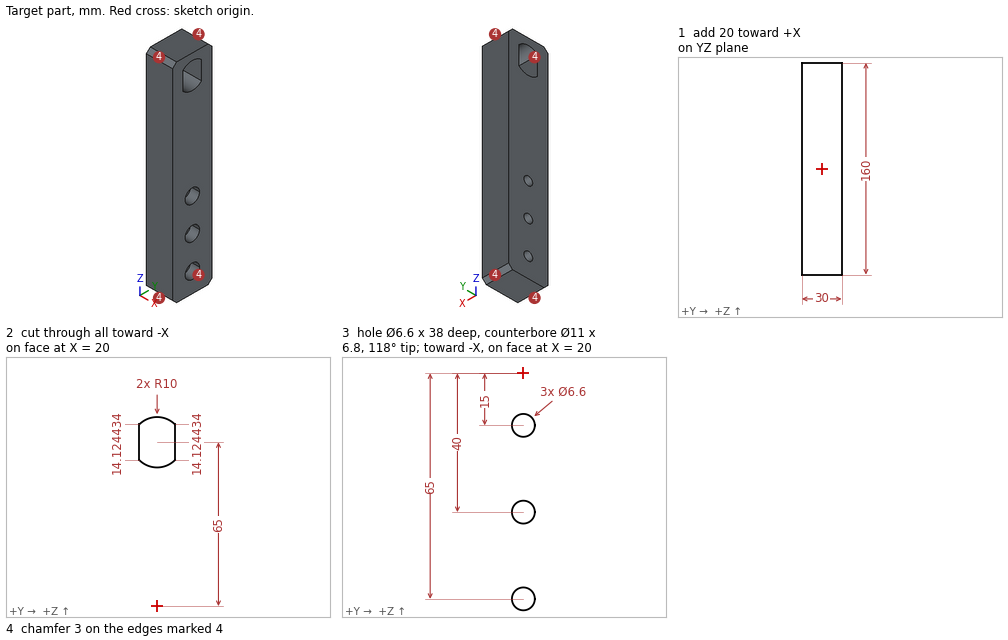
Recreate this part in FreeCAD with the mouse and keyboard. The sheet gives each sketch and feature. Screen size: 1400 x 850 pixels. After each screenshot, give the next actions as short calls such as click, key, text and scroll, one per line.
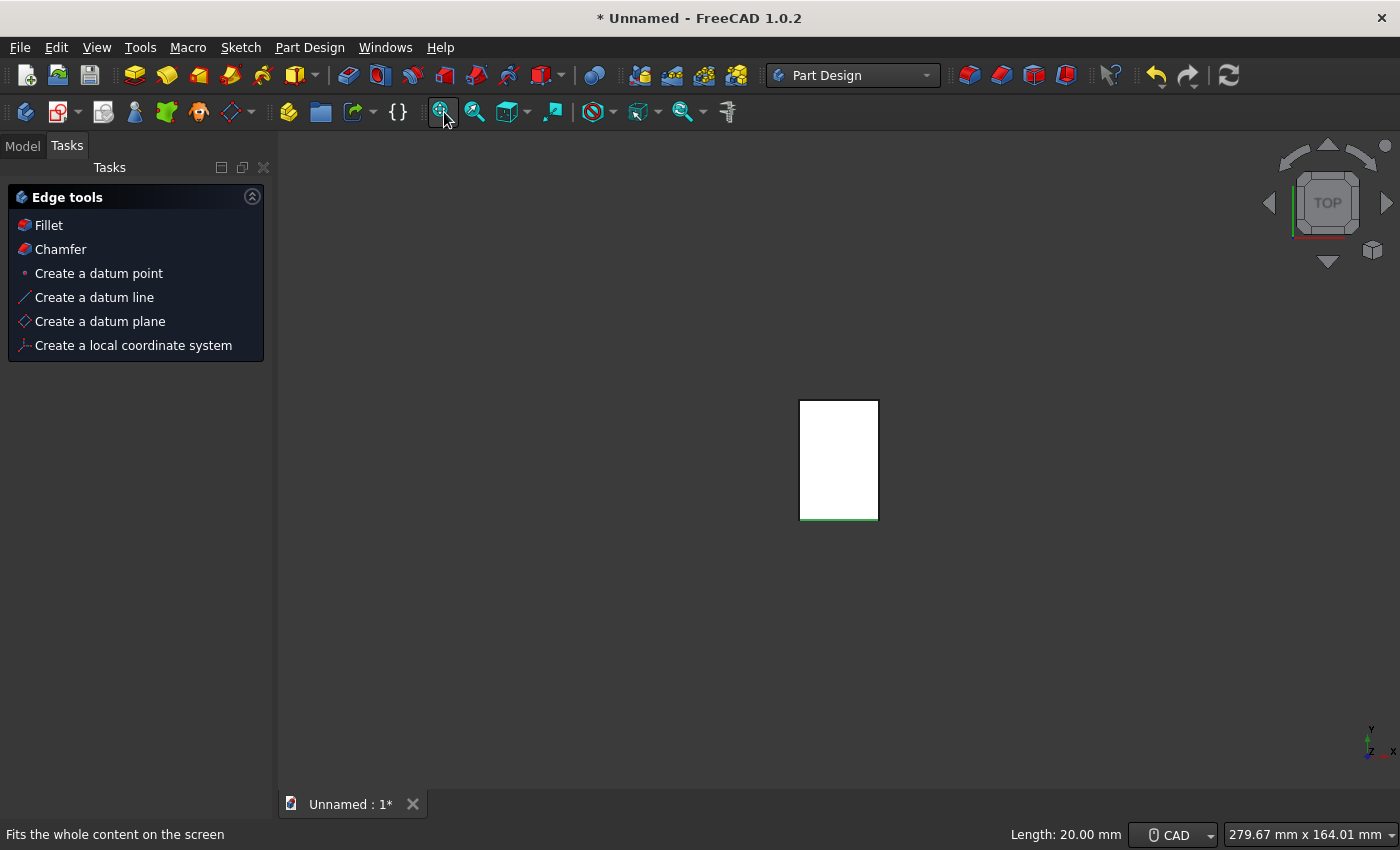
click(839, 399, ctrl)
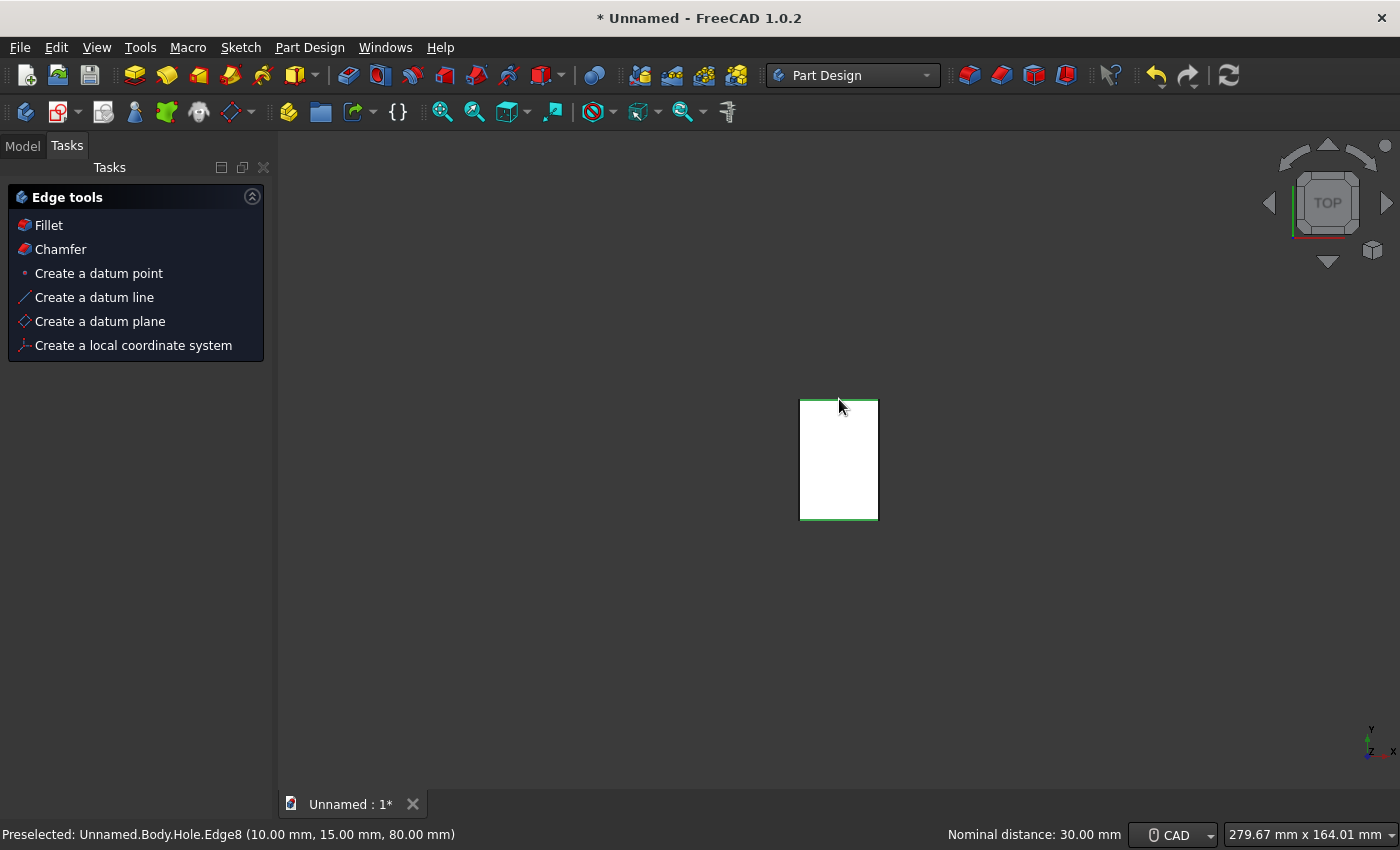
key(1)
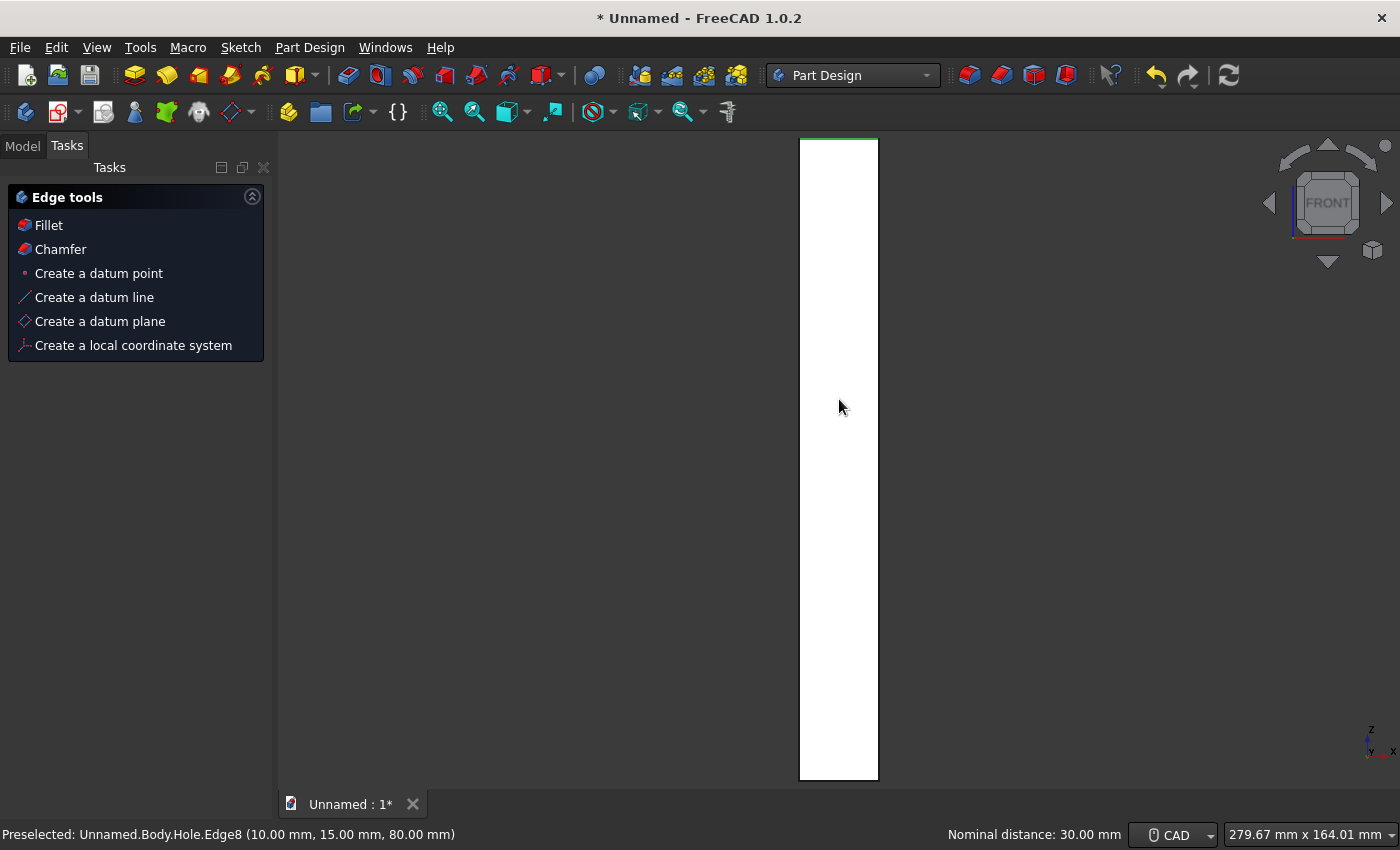
key(3)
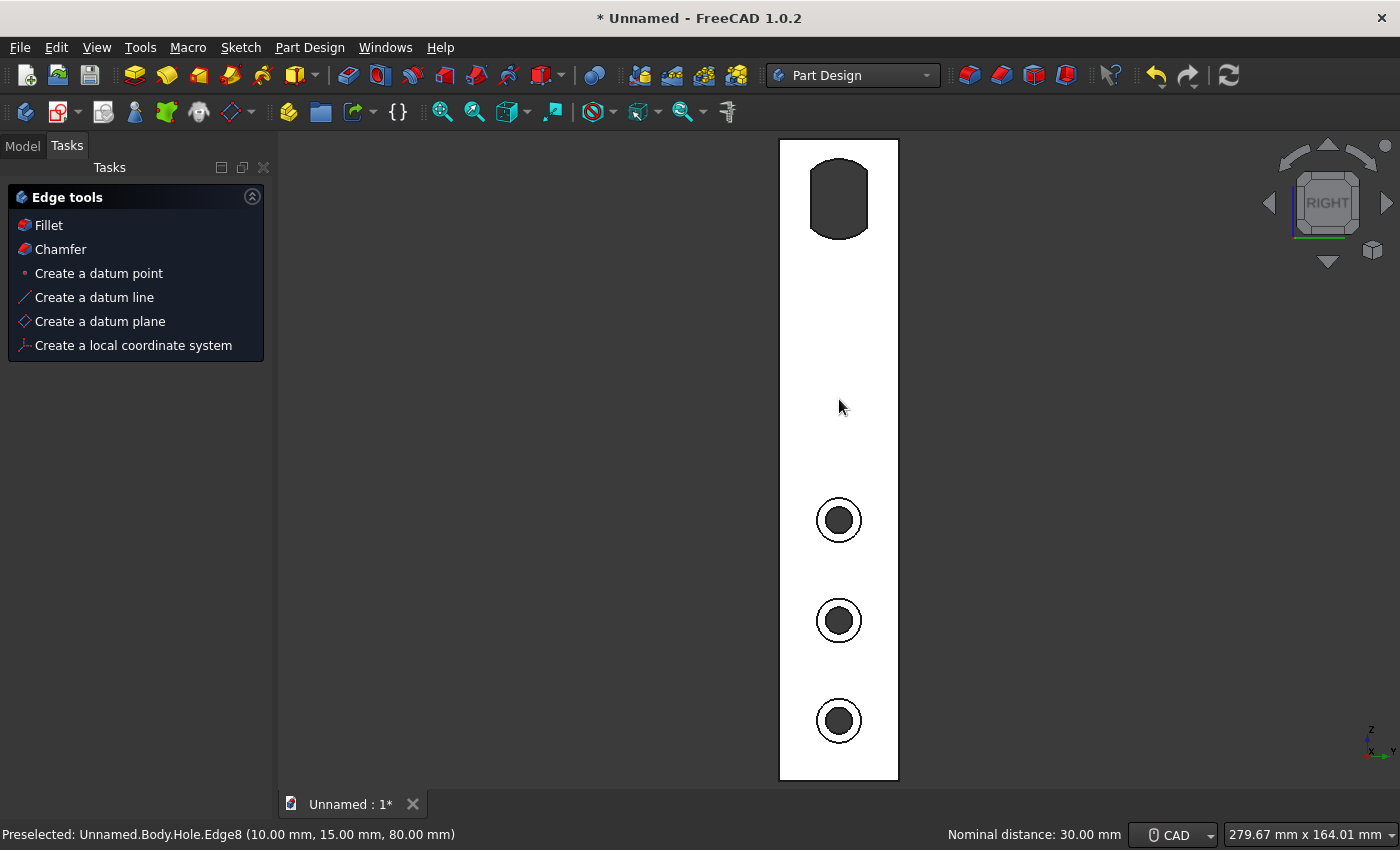
key(5)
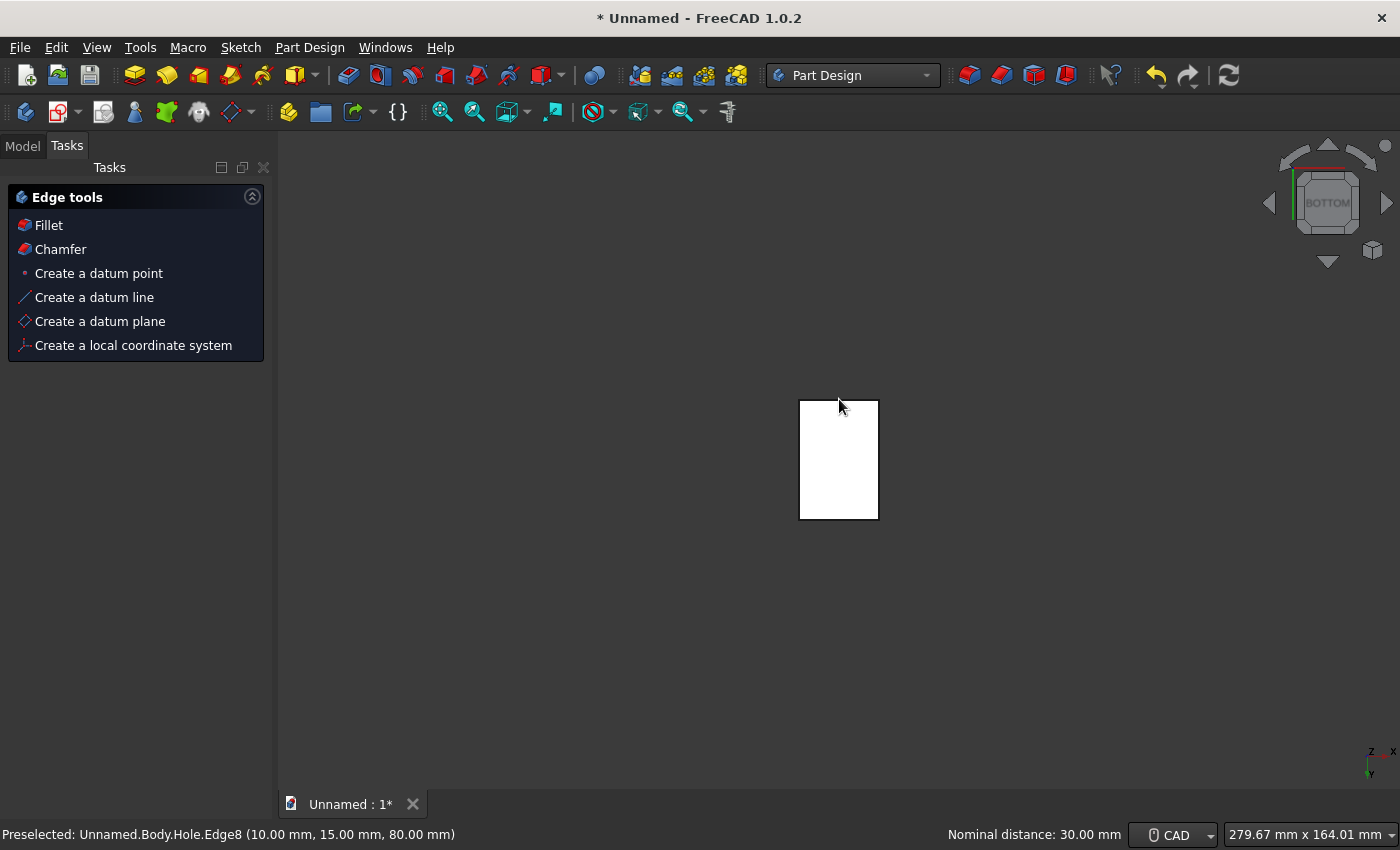
key(v)
key(f)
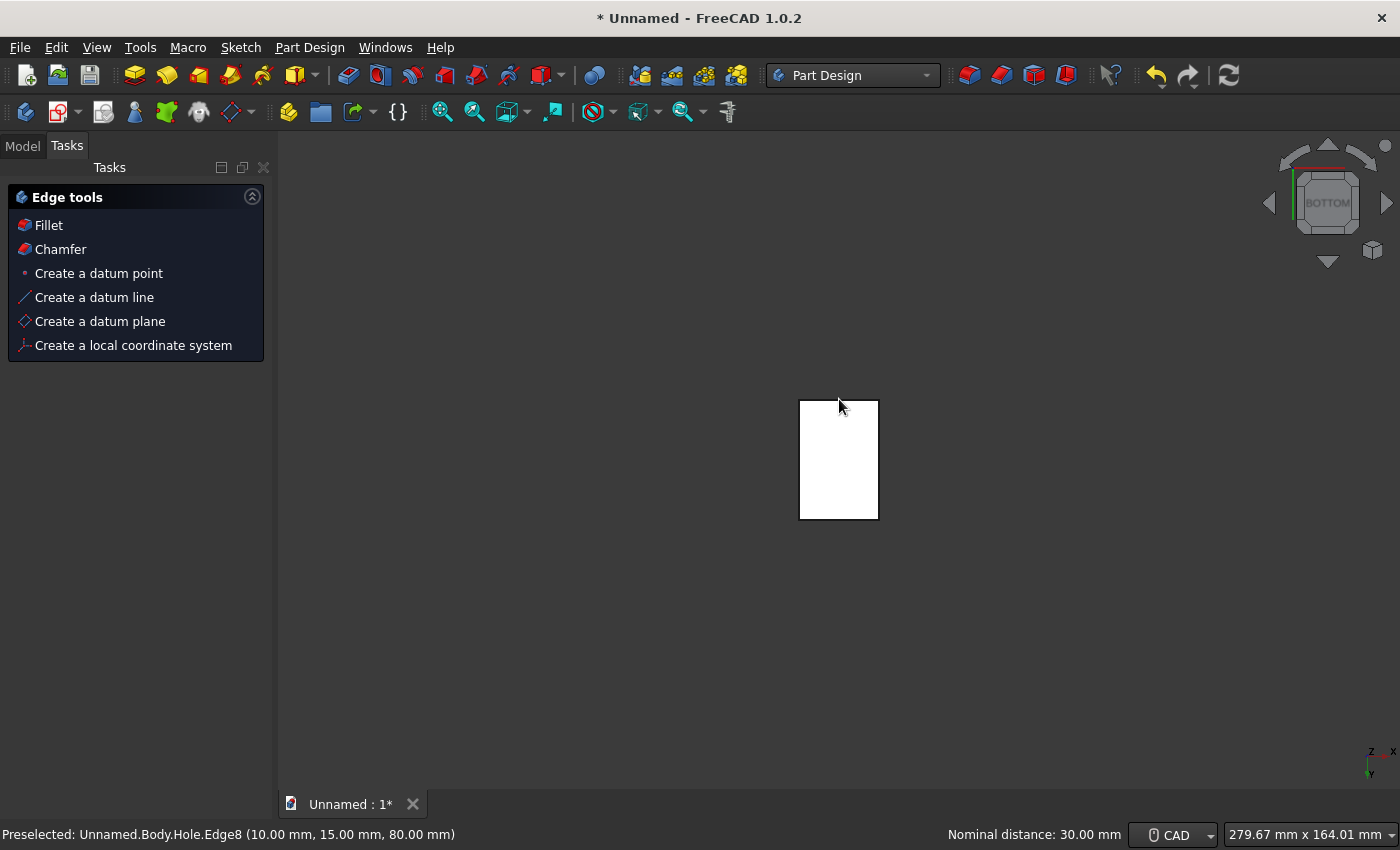
click(839, 399, ctrl)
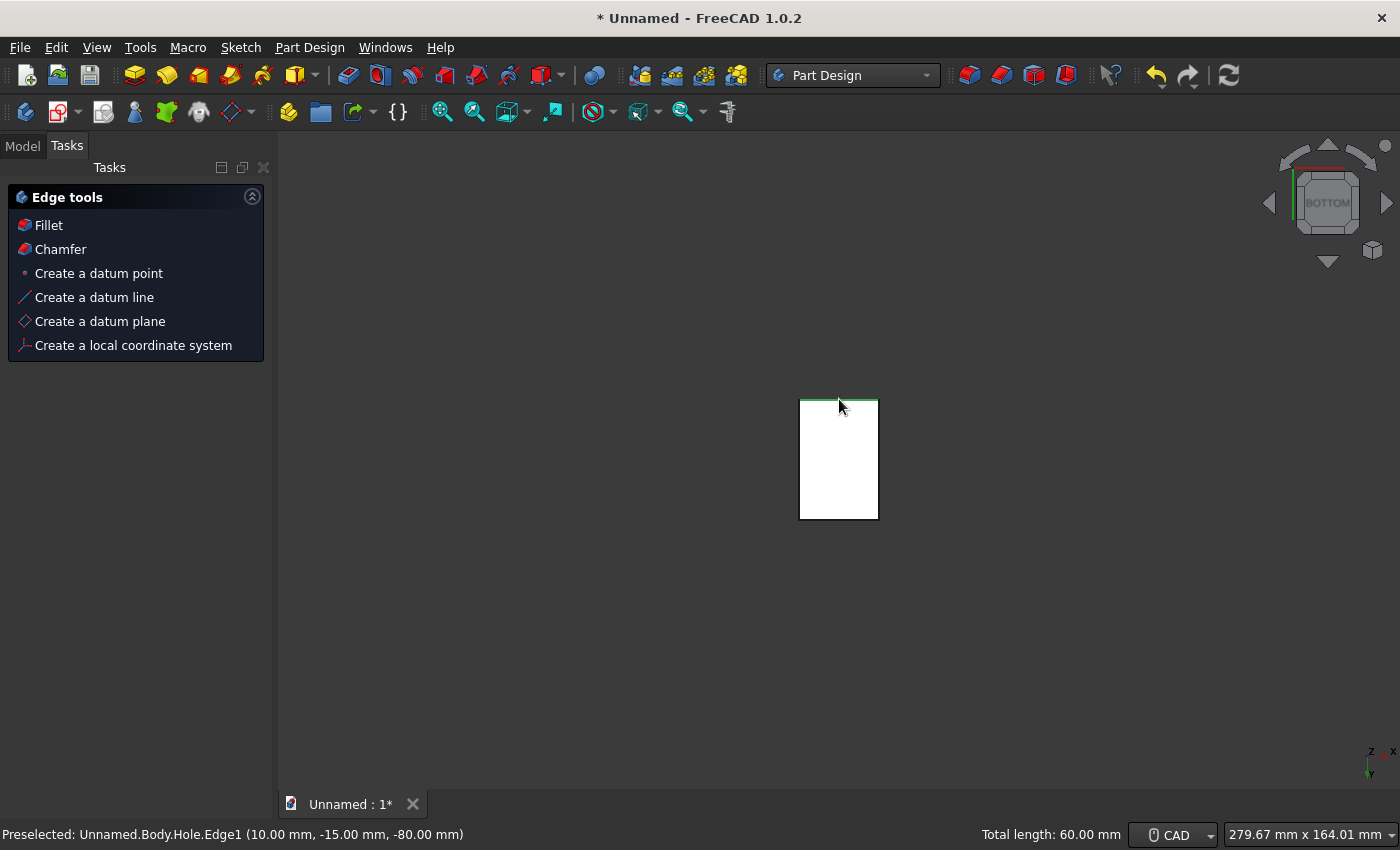
click(839, 519, ctrl)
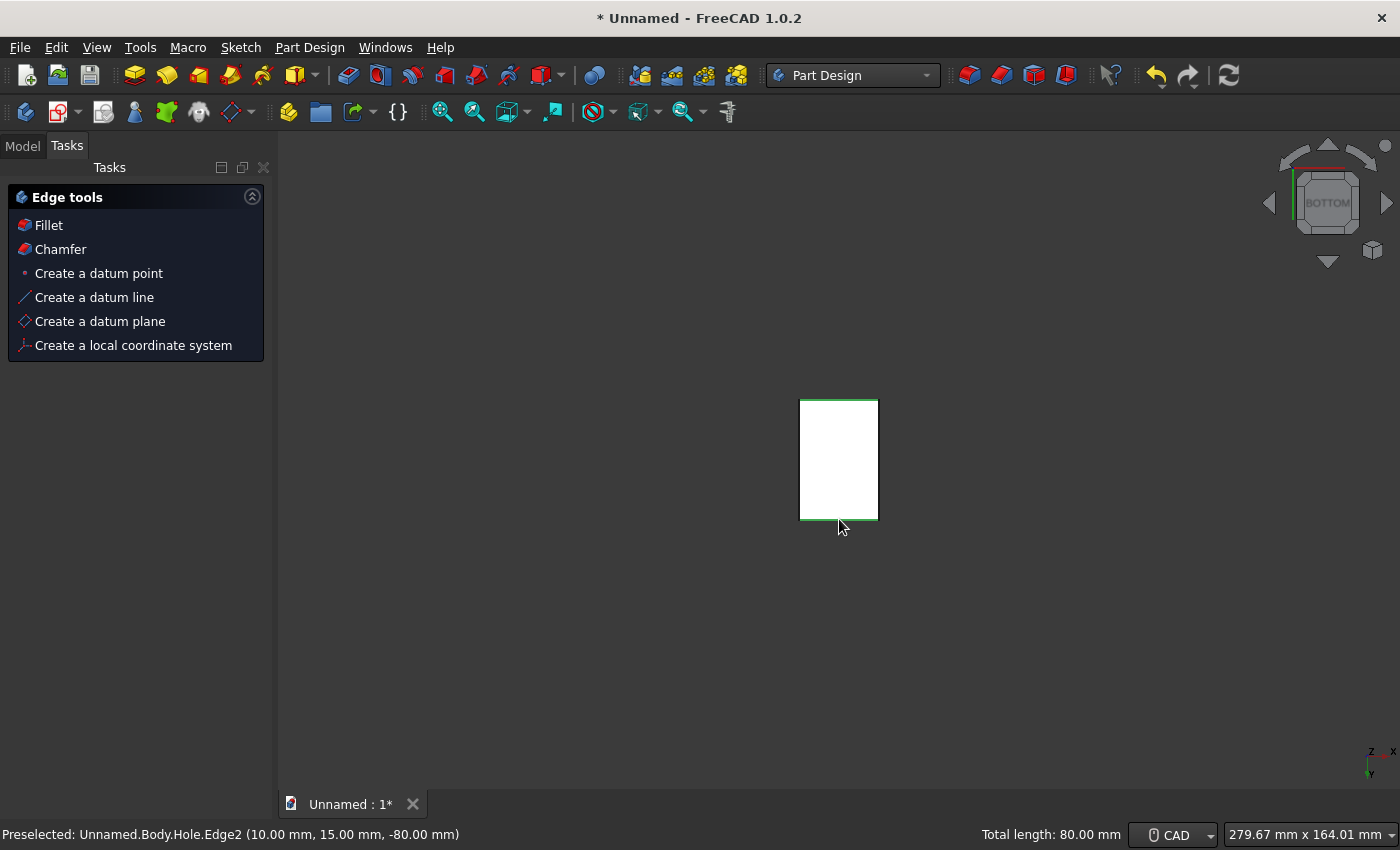
click(1002, 76)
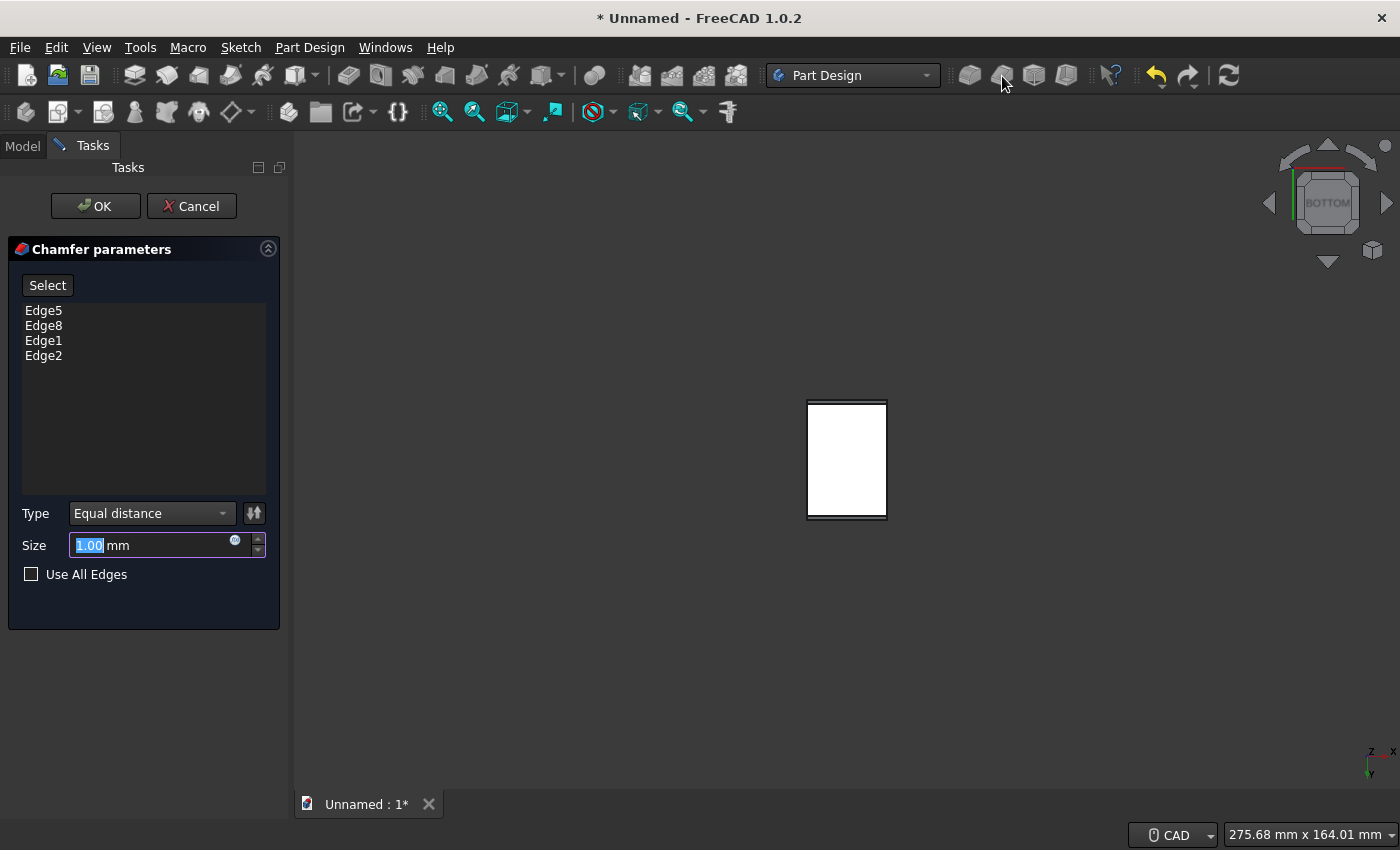
text(3)
key(Tab)